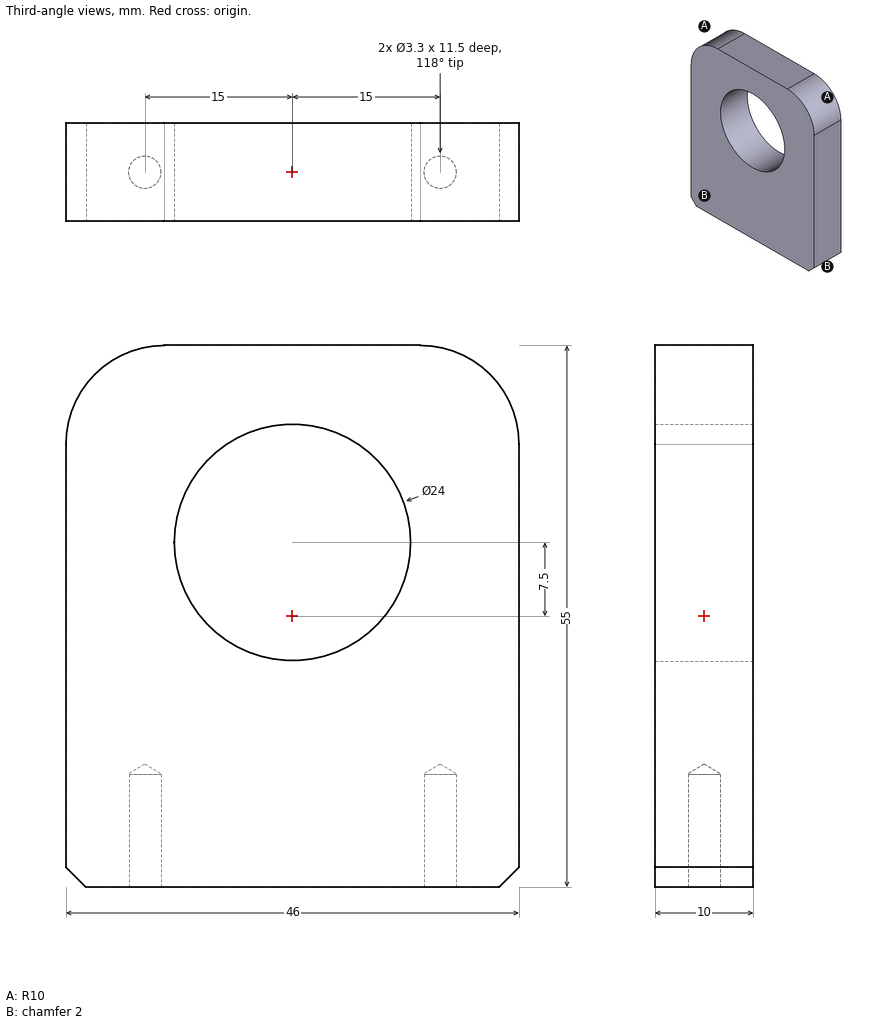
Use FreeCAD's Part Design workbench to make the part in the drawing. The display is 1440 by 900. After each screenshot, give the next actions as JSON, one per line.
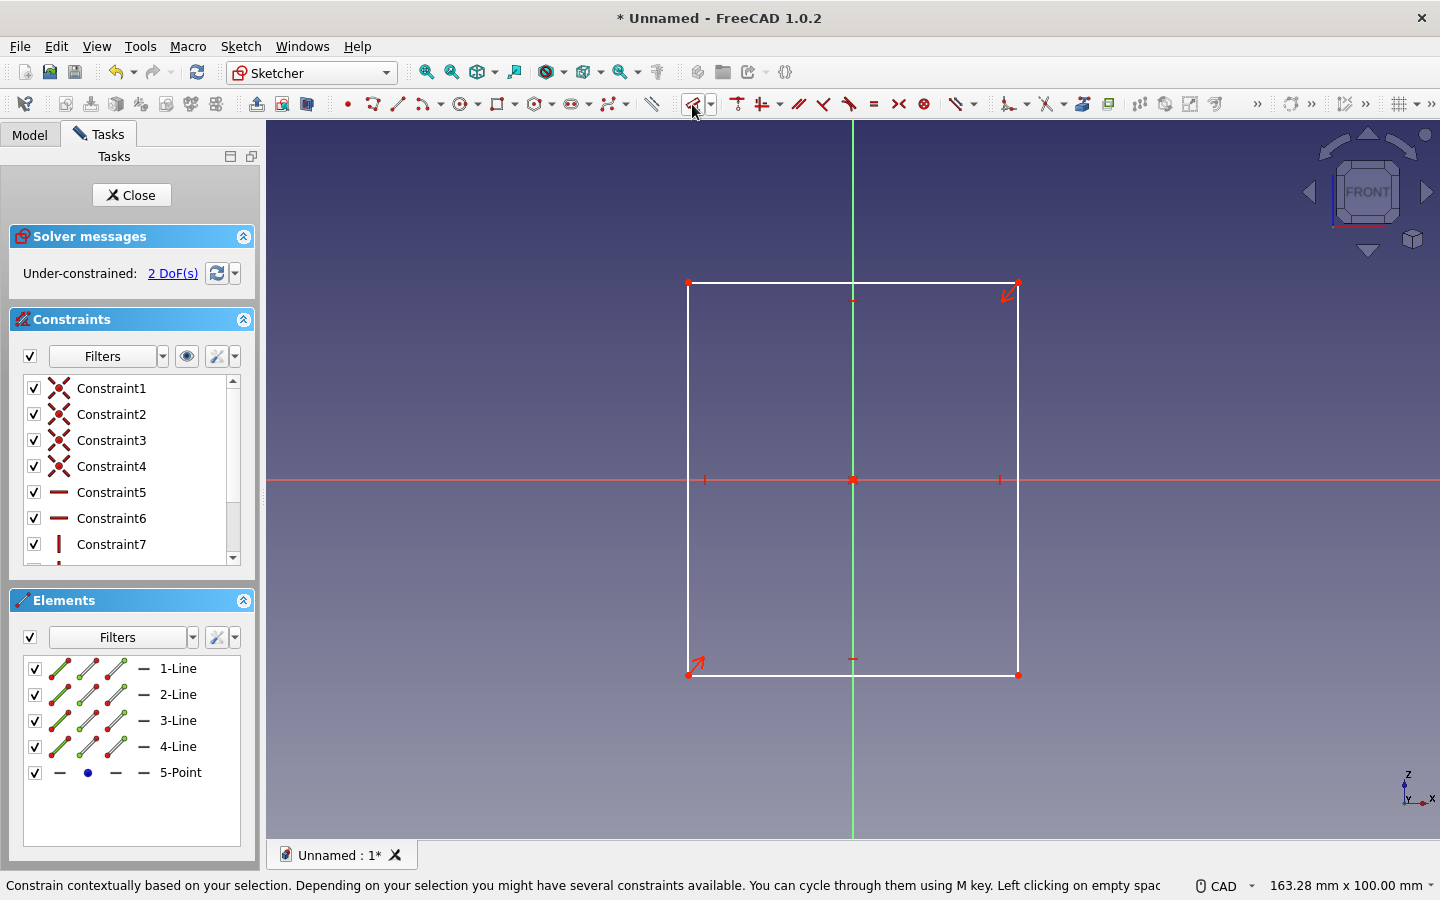
{"action": "left_click", "coordinate": [787, 676]}
{"action": "left_click", "coordinate": [777, 710]}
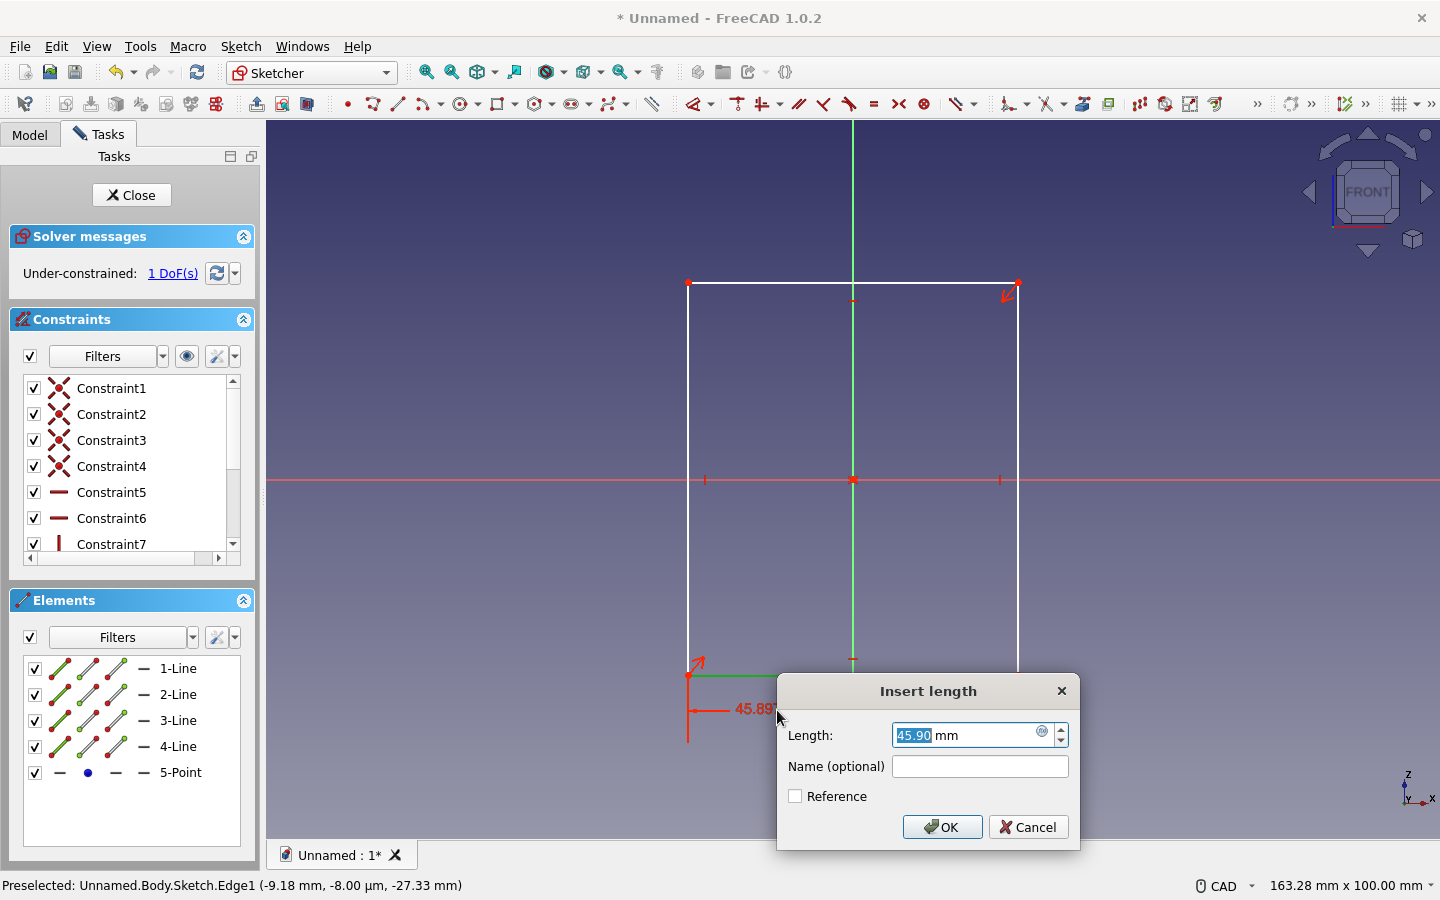
{"action": "type", "text": "46"}
{"action": "key", "text": "Return"}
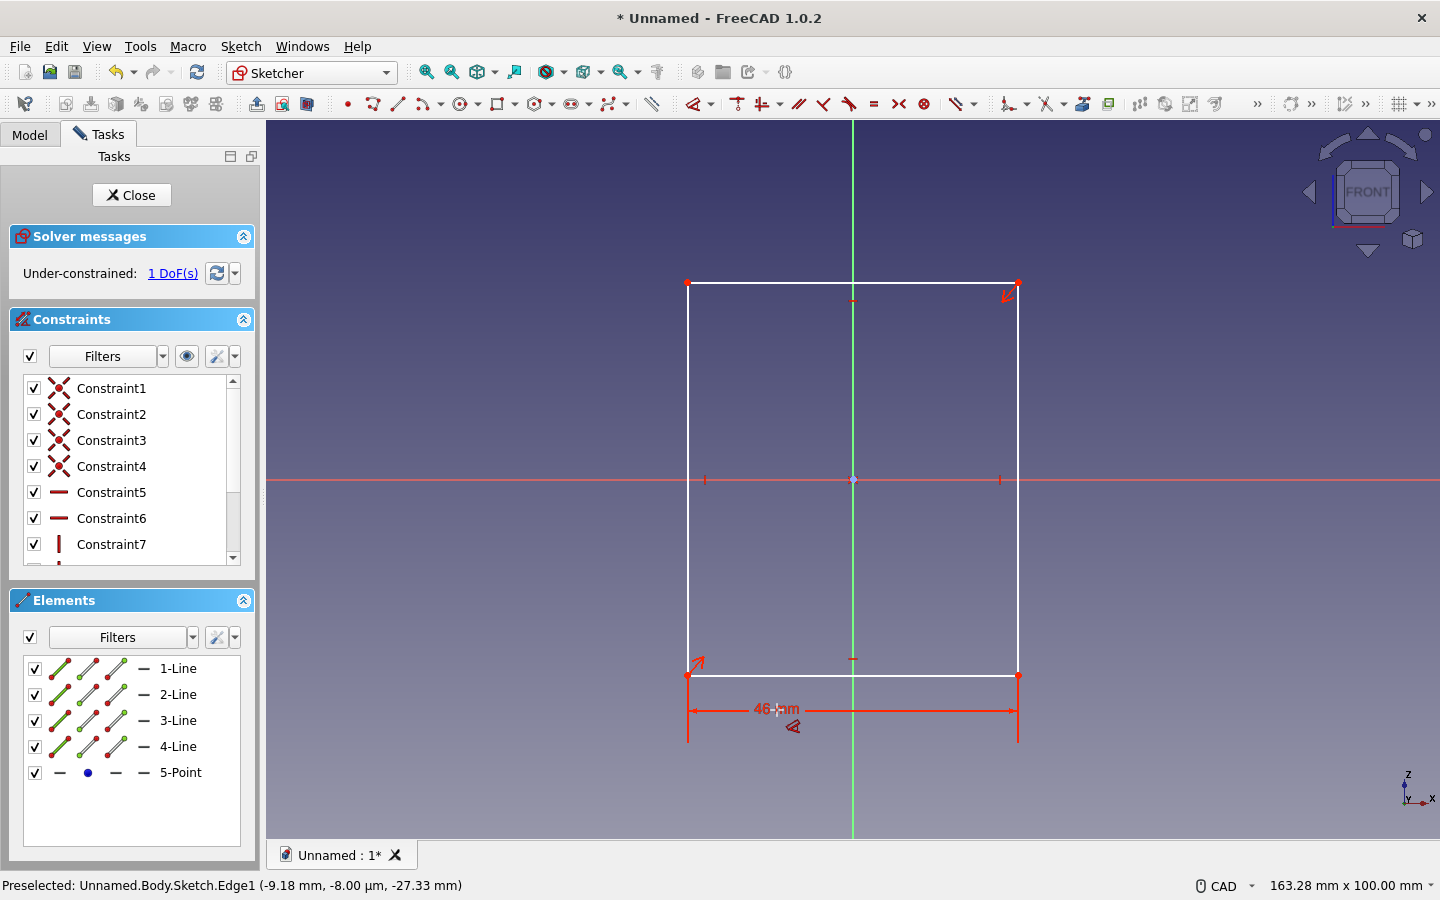
{"action": "left_click", "coordinate": [1018, 558]}
{"action": "left_click", "coordinate": [1052, 389]}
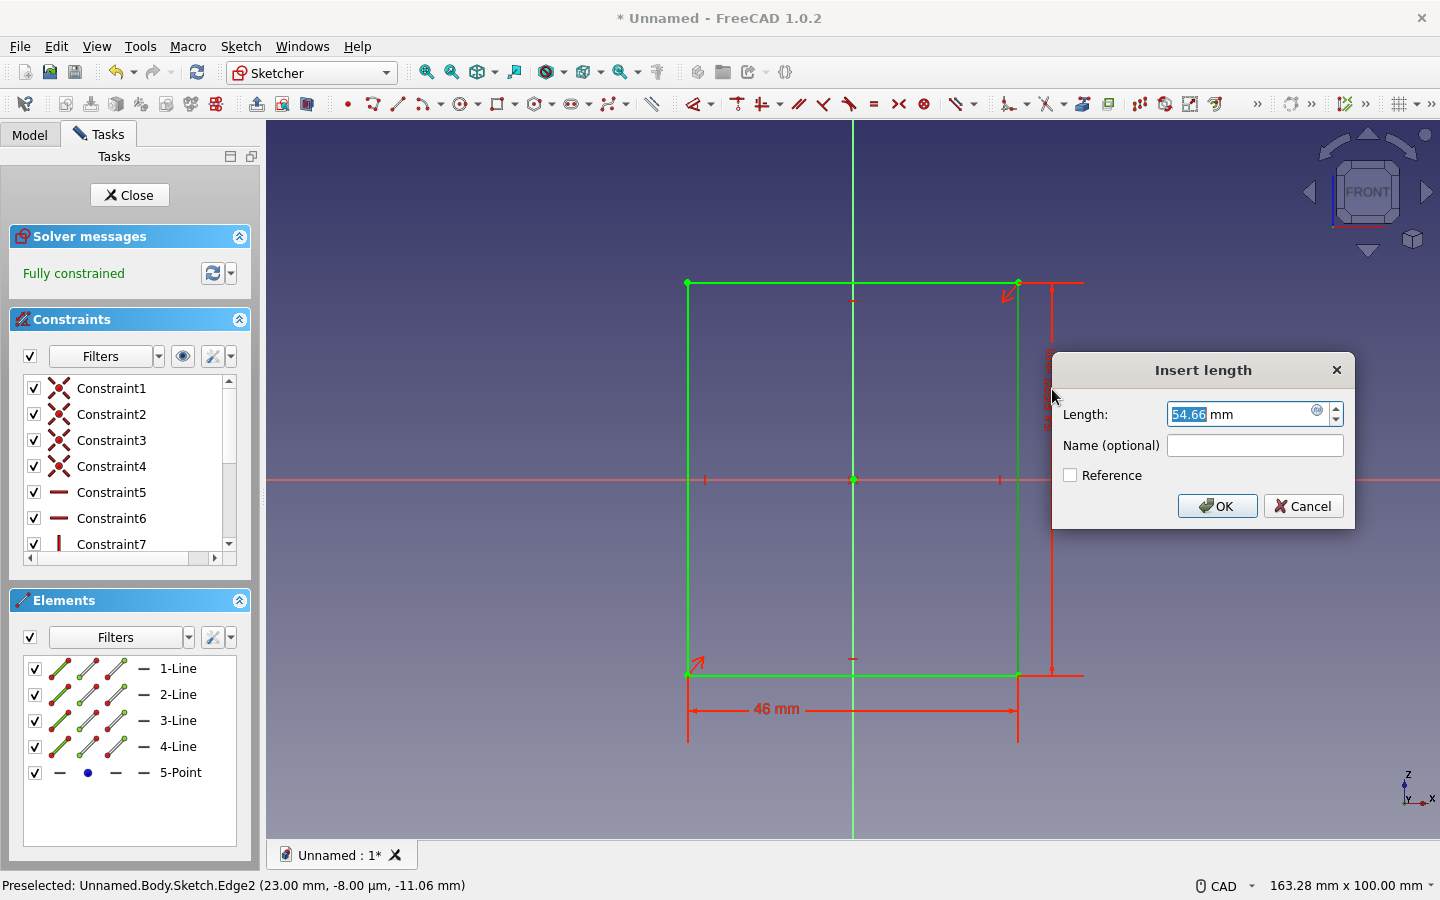
{"action": "type", "text": "55"}
{"action": "key", "text": "Return"}
{"action": "key", "text": "Escape"}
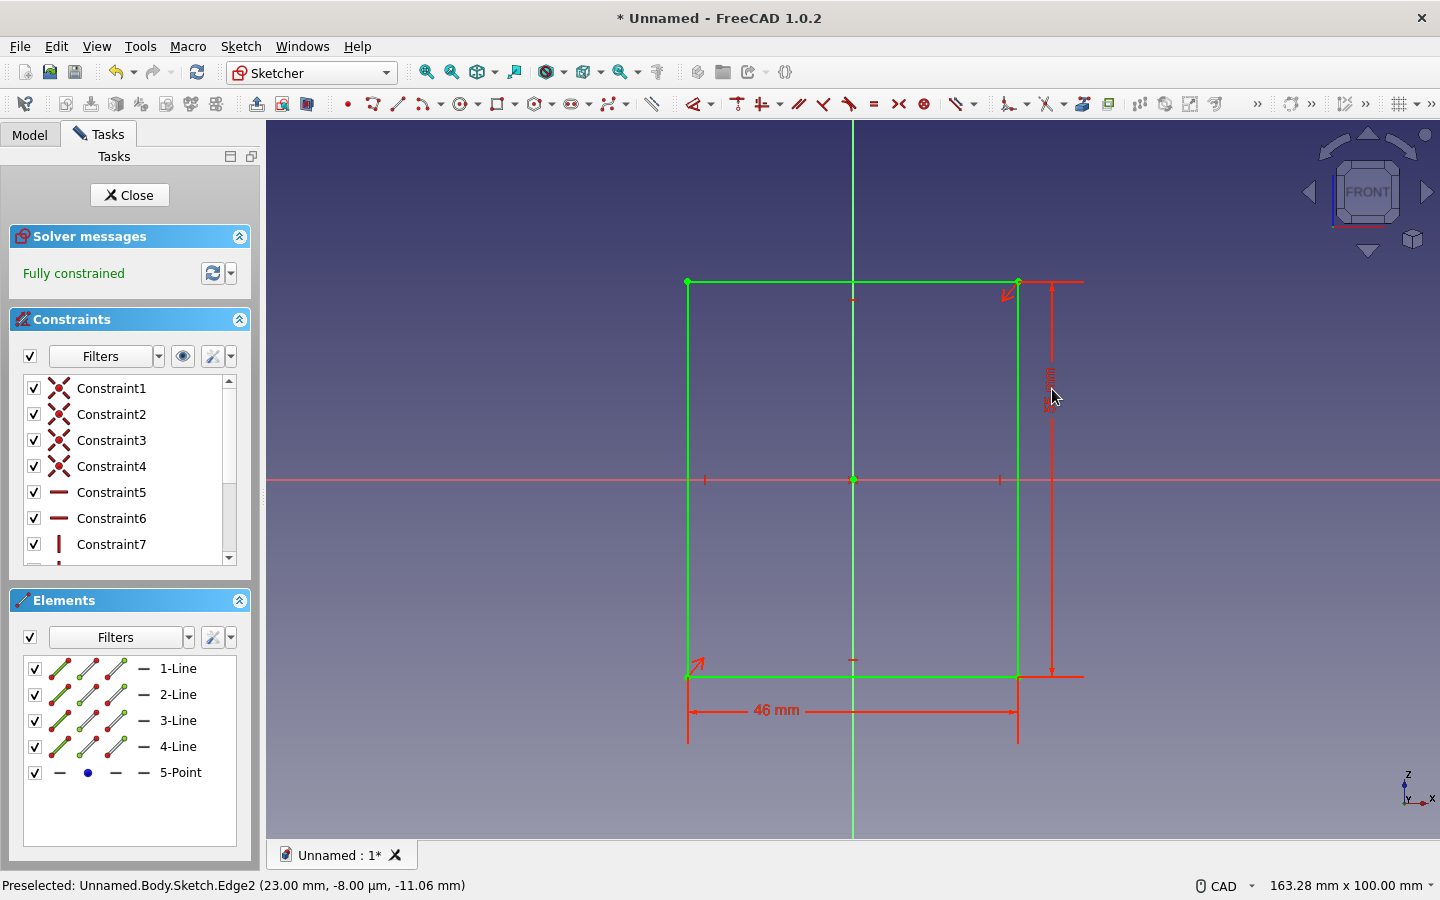
{"action": "left_click", "coordinate": [130, 195]}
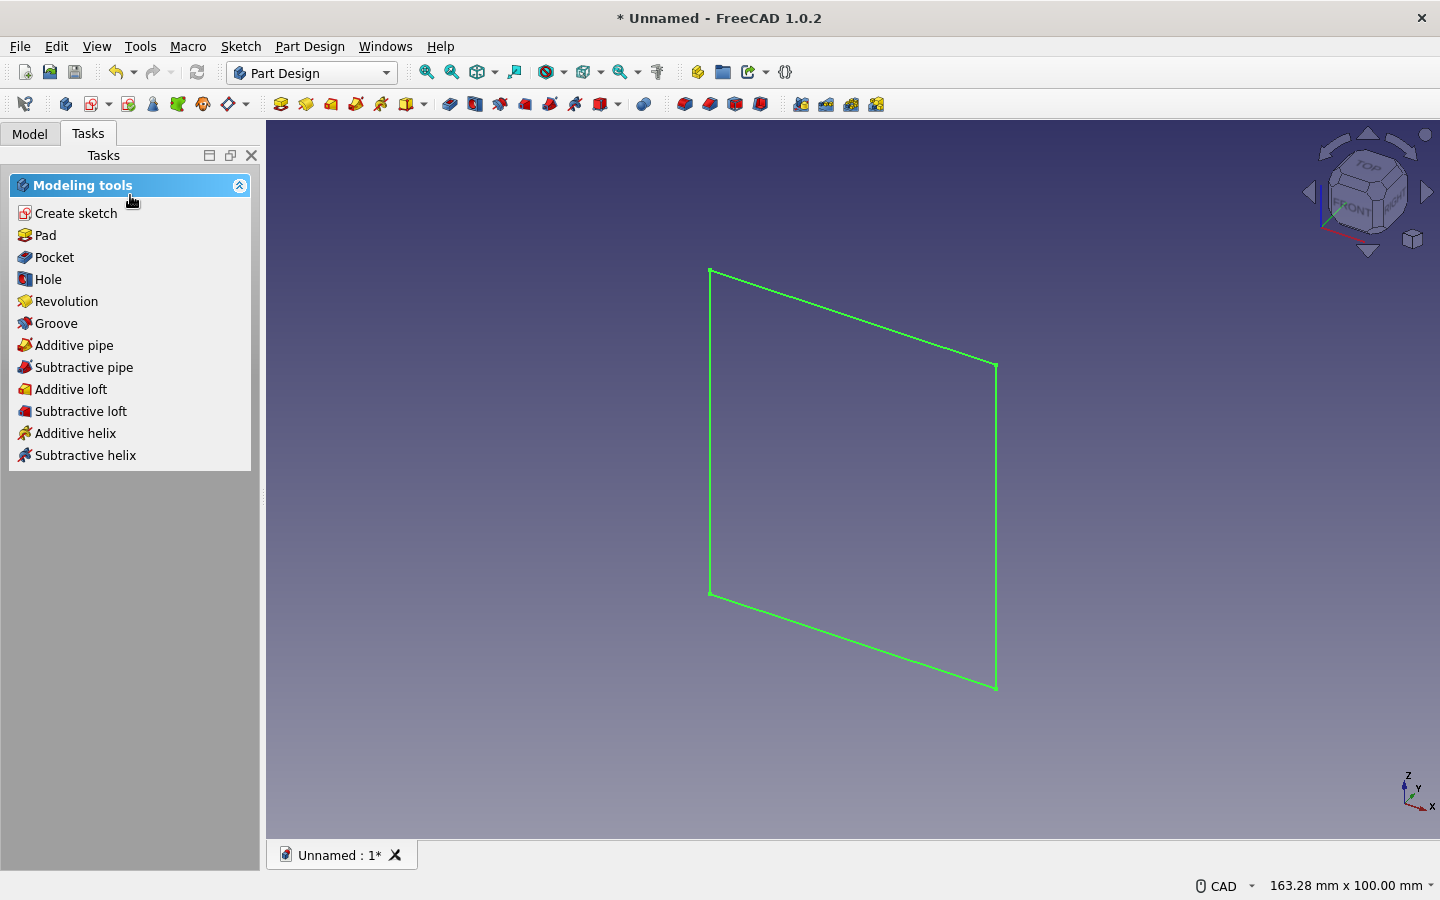
{"action": "left_click", "coordinate": [281, 104]}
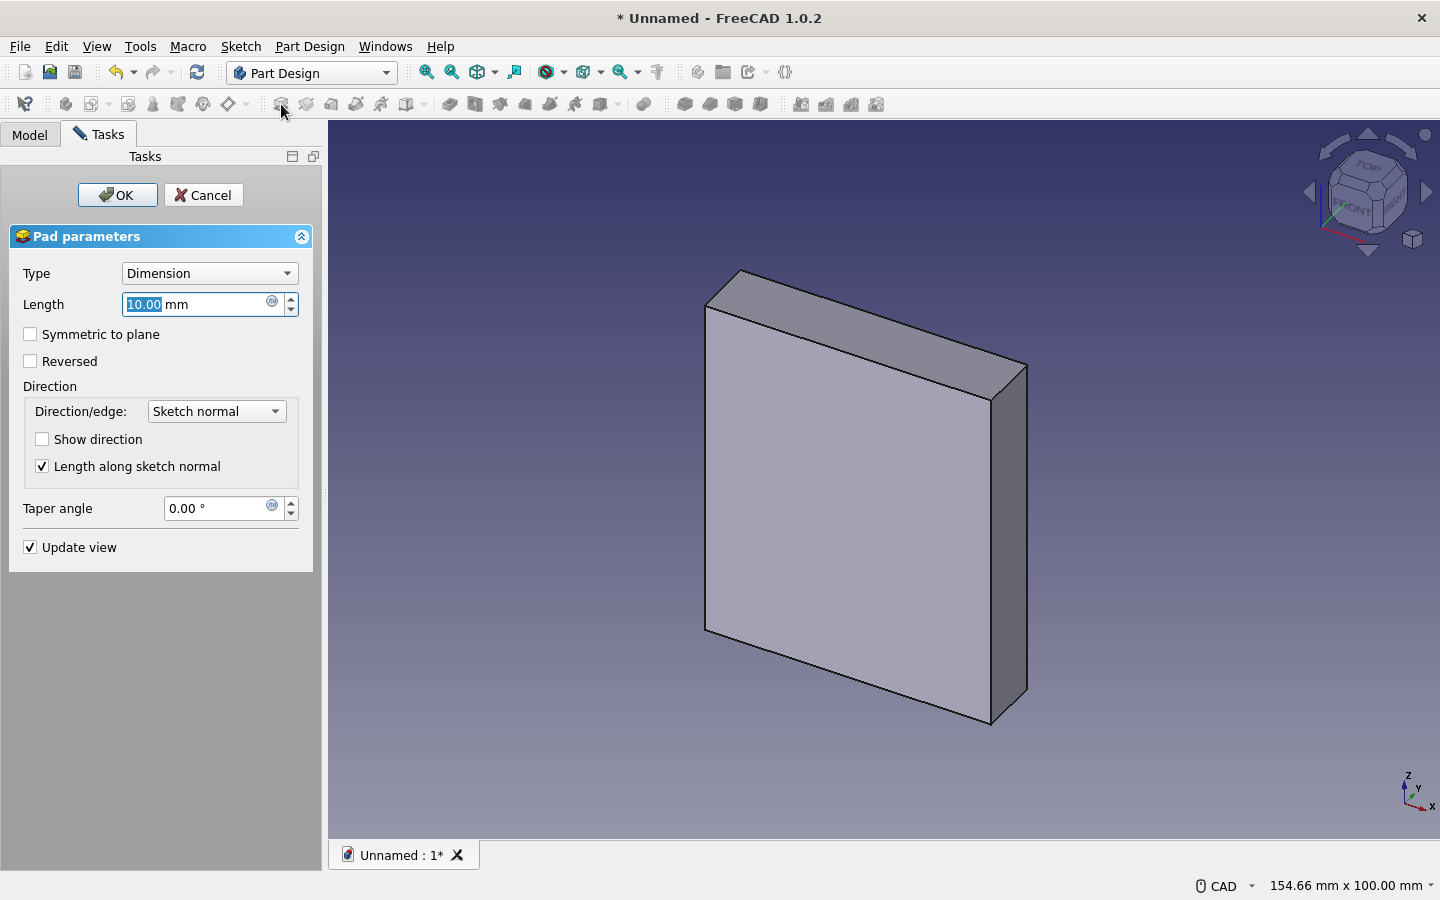
{"action": "type", "text": "10"}
{"action": "key", "text": "Tab"}